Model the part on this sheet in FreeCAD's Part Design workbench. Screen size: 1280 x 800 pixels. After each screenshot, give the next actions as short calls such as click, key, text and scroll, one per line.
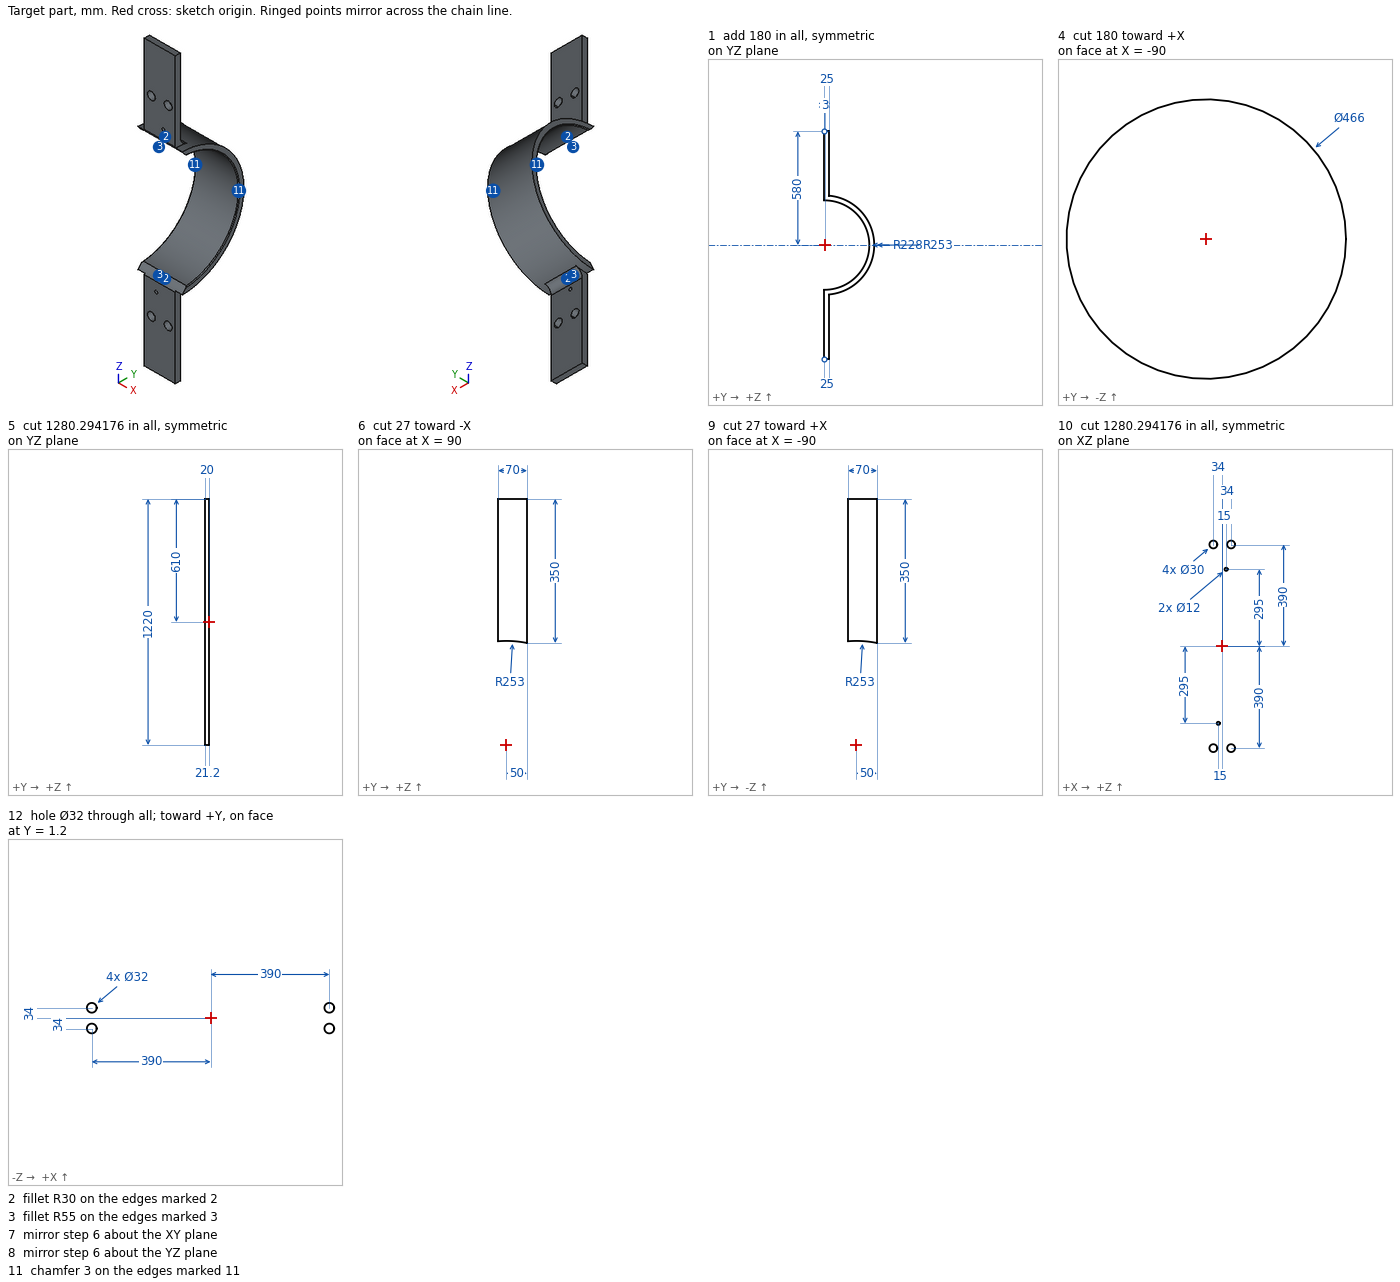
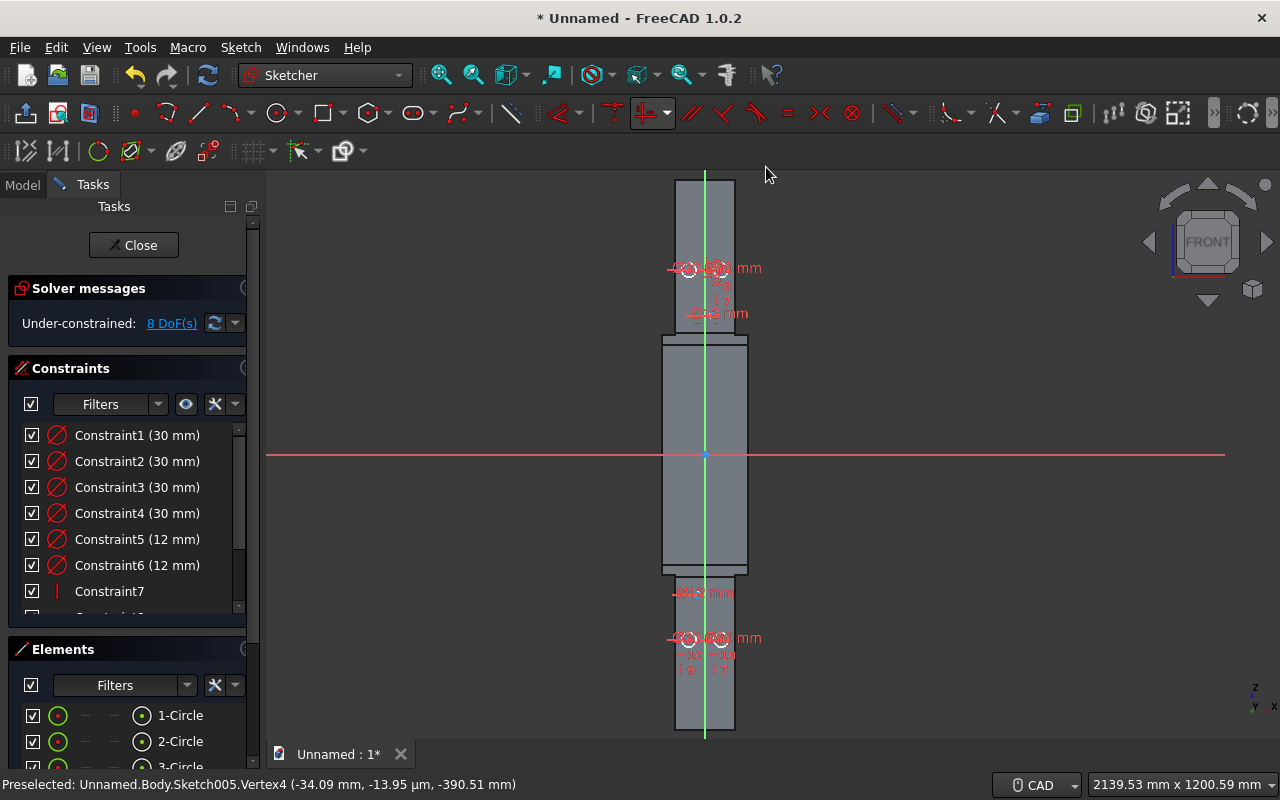
click(558, 114)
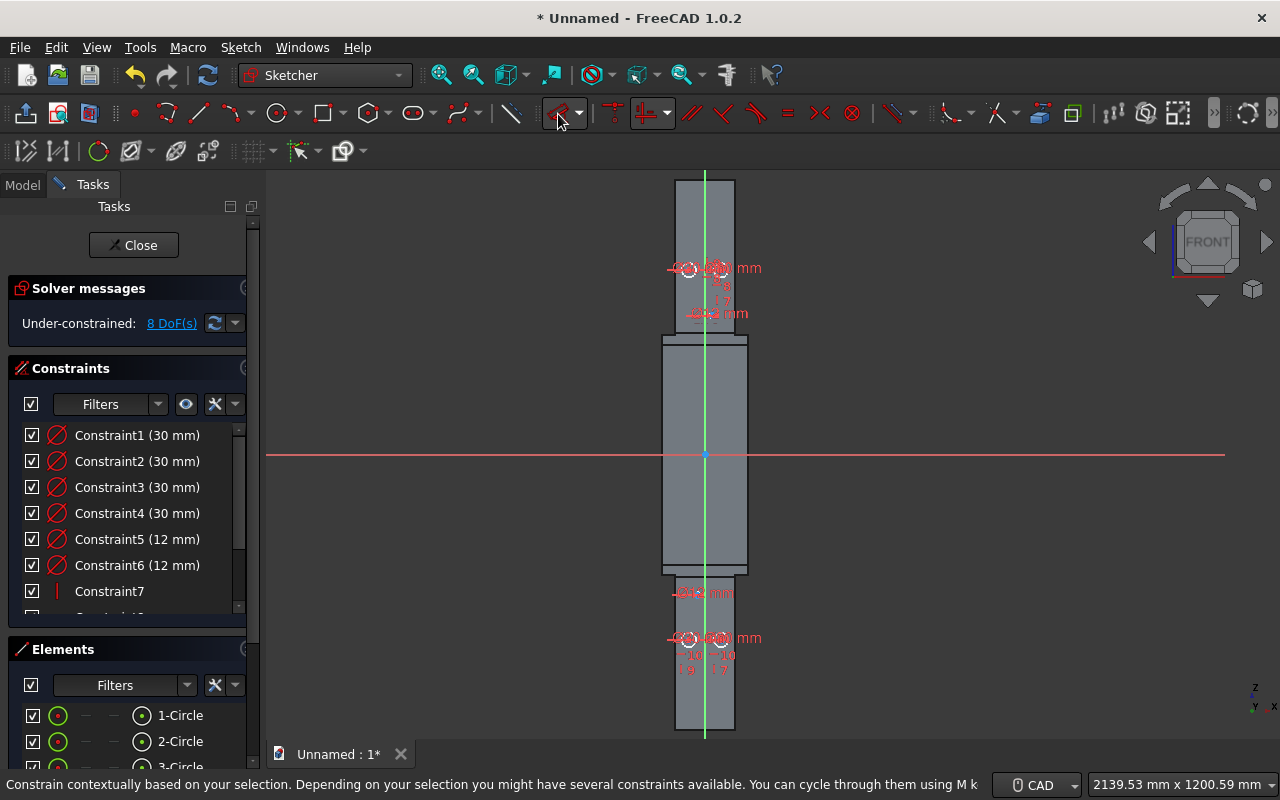
scroll(721, 270, up, 5)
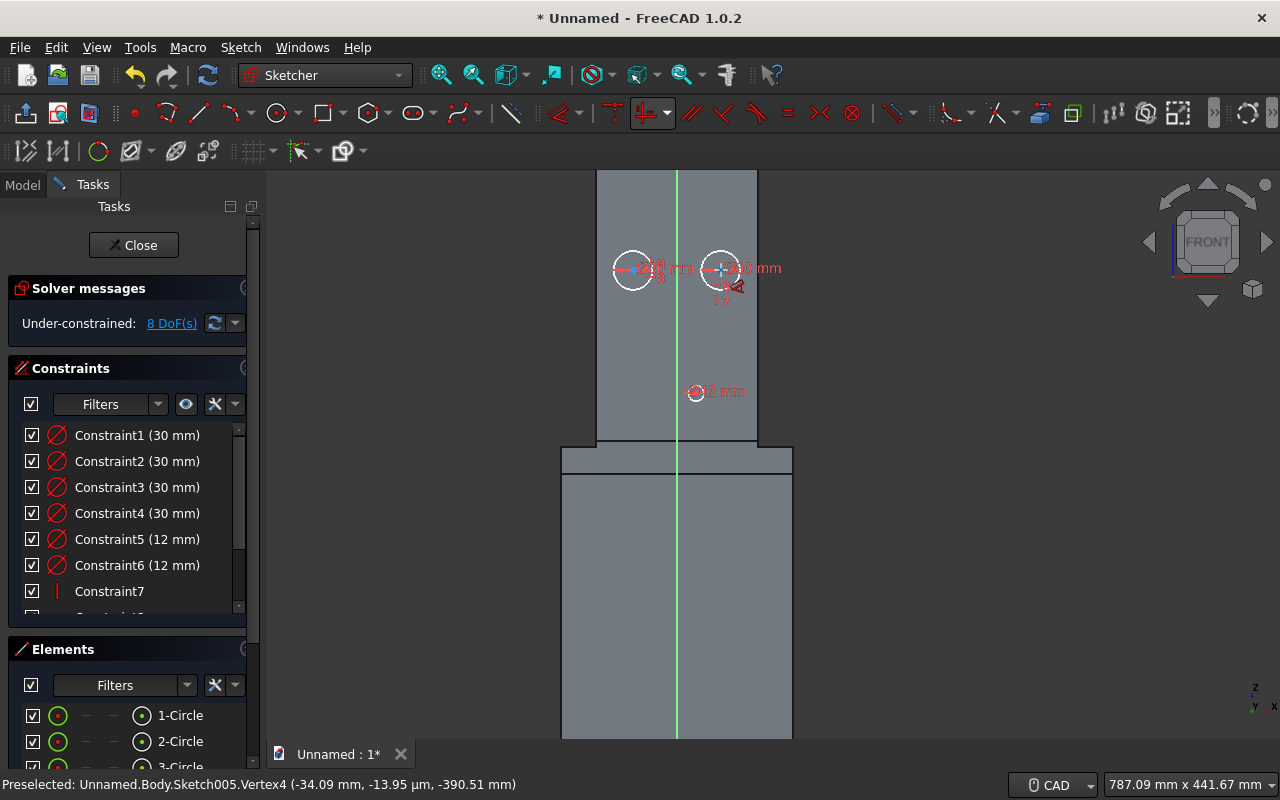
click(721, 270)
click(699, 236)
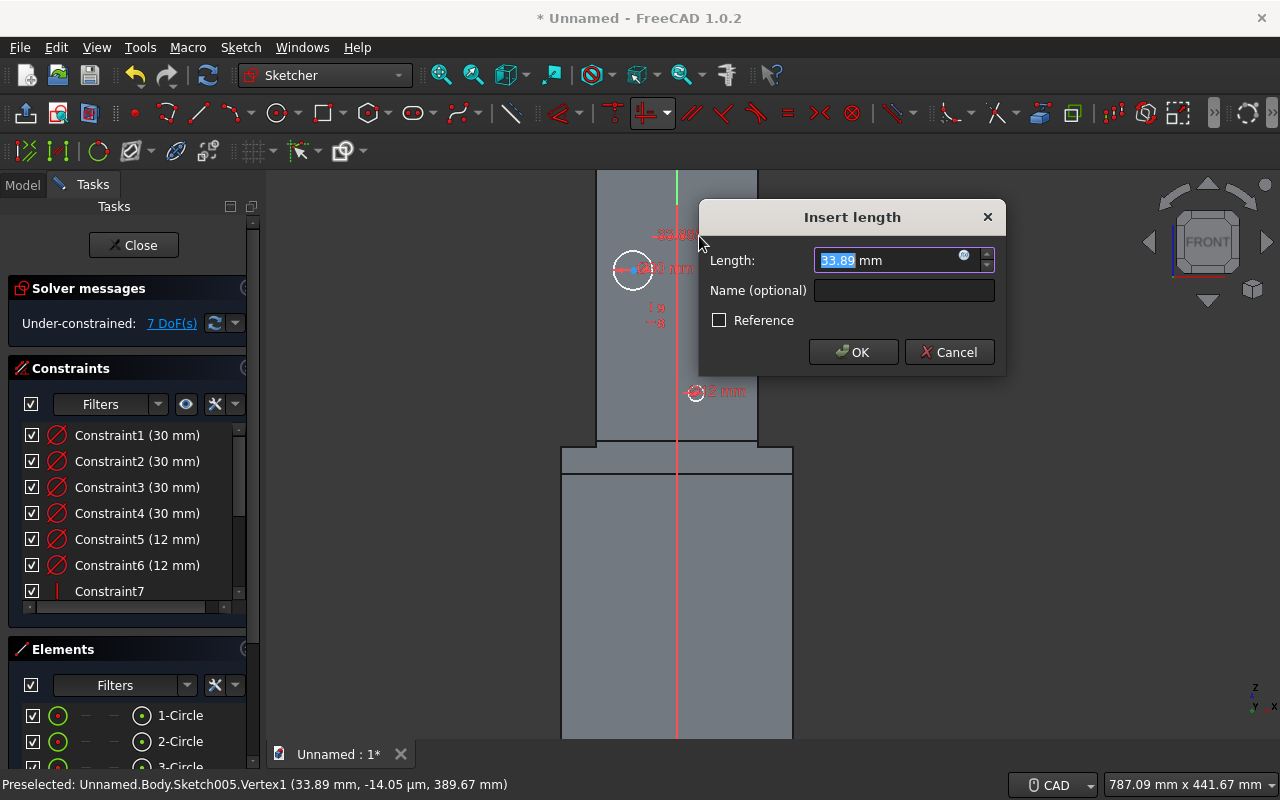
text(34)
key(Return)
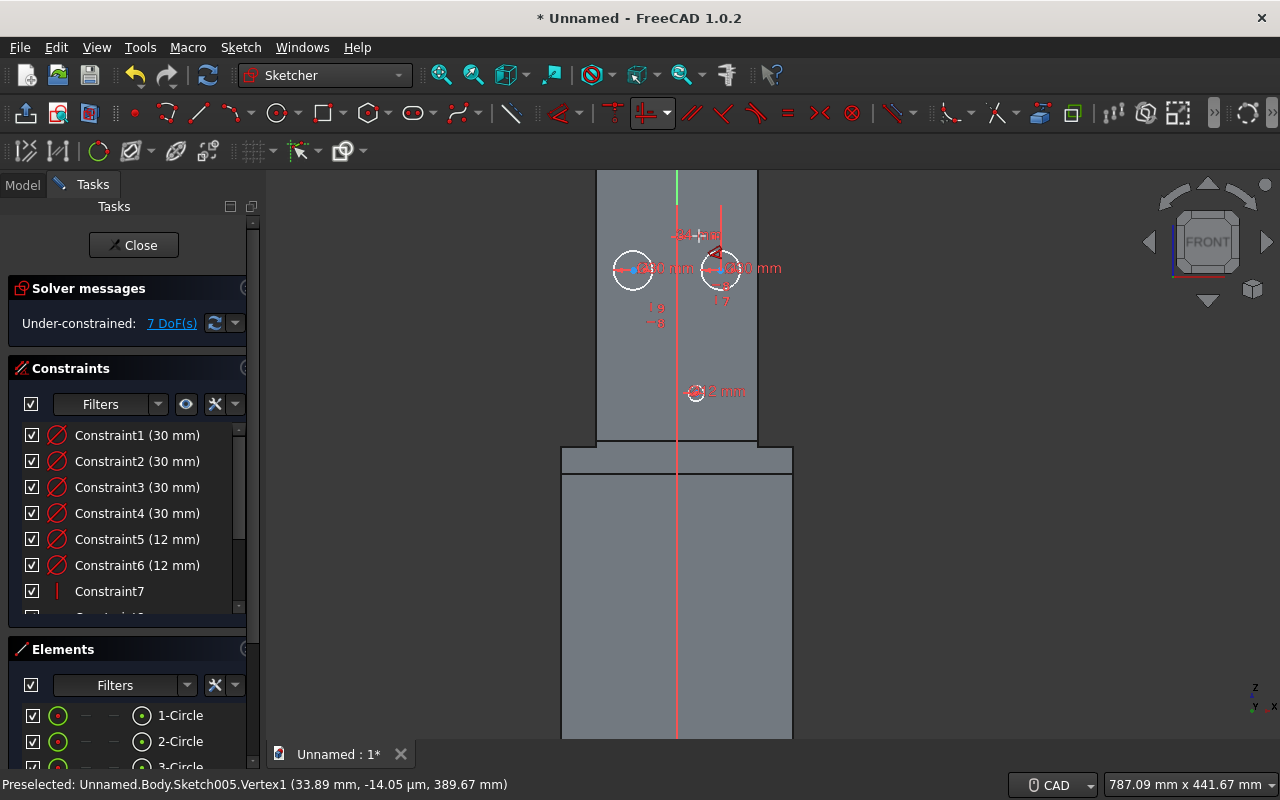
click(633, 270)
click(655, 212)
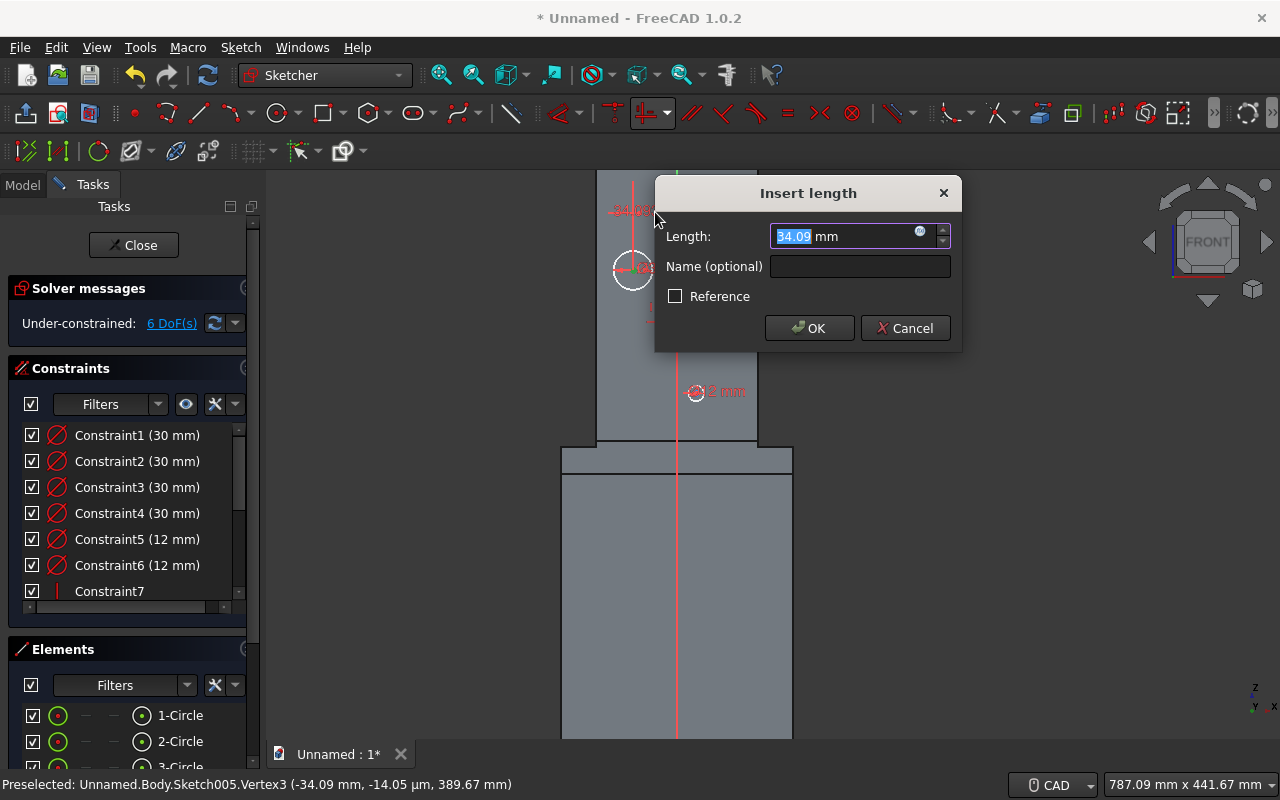
text(34)
key(Return)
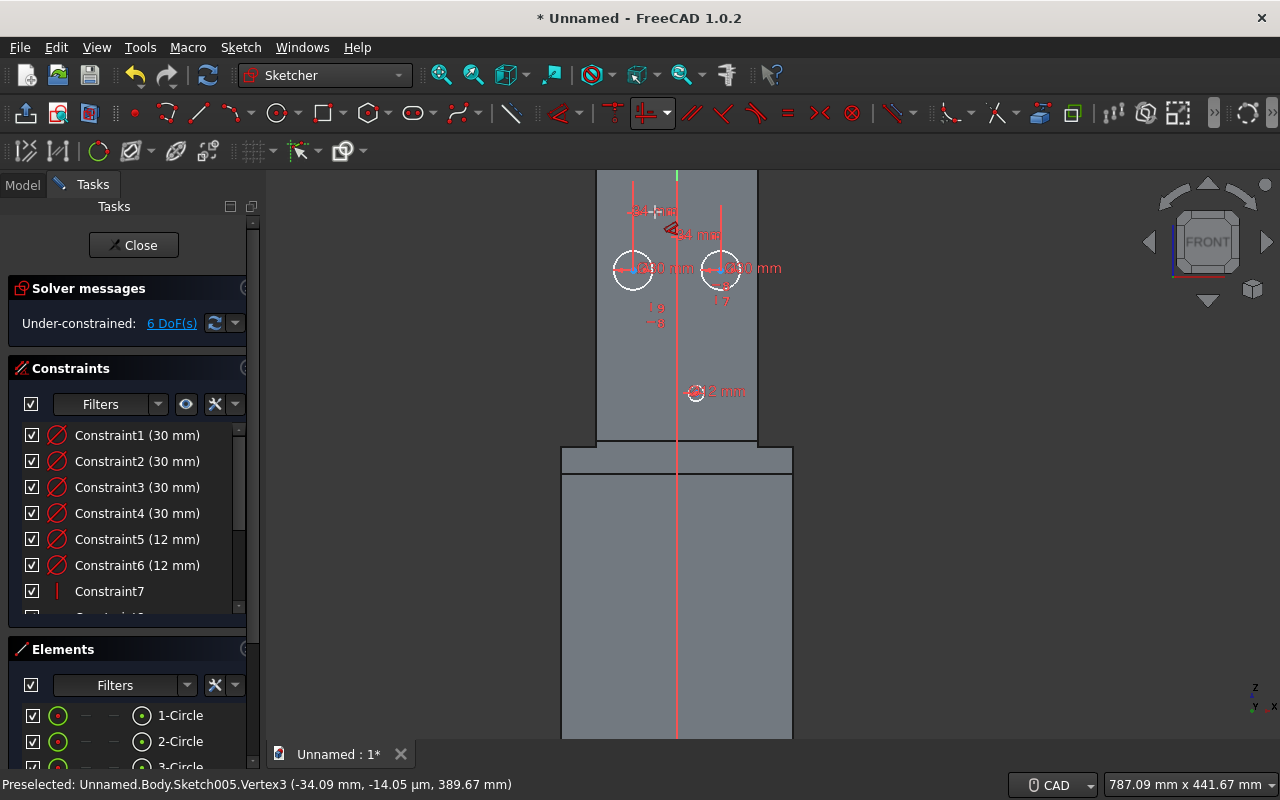
scroll(696, 393, up, 4)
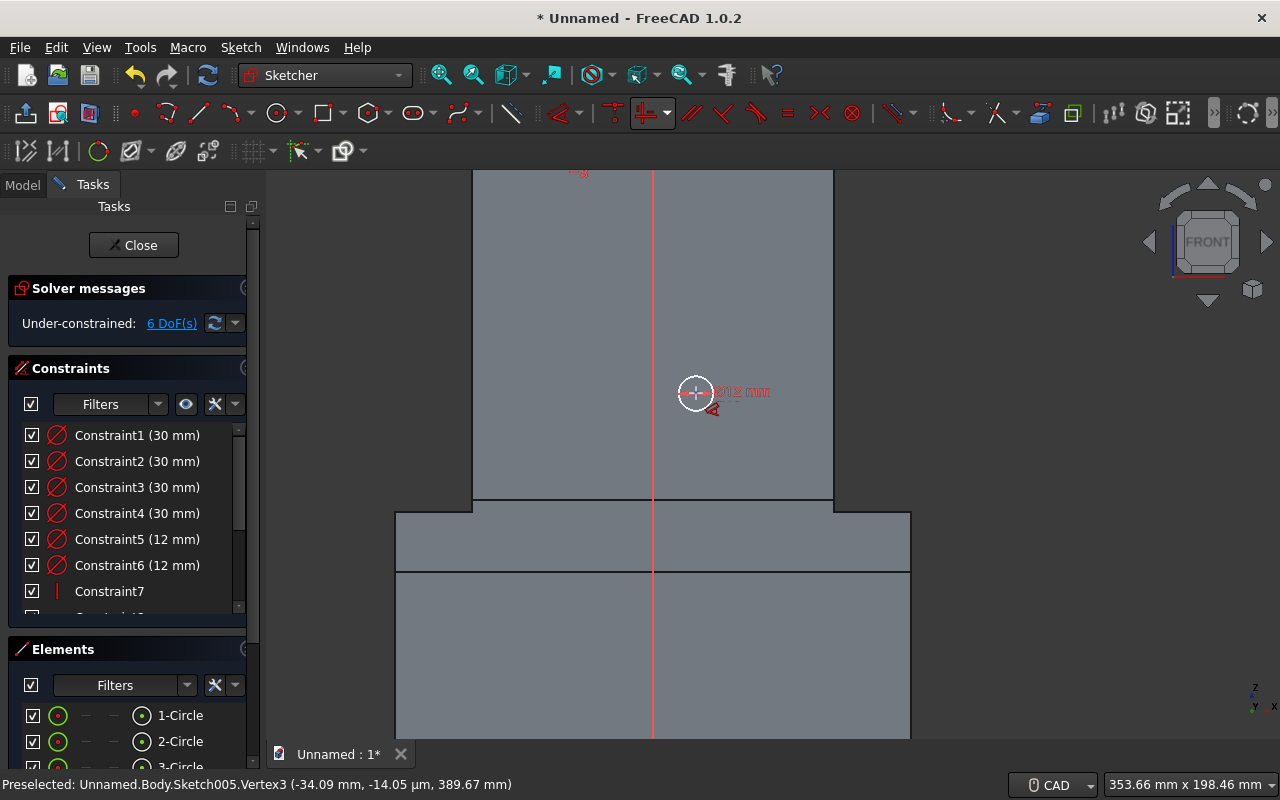
click(696, 394)
click(675, 360)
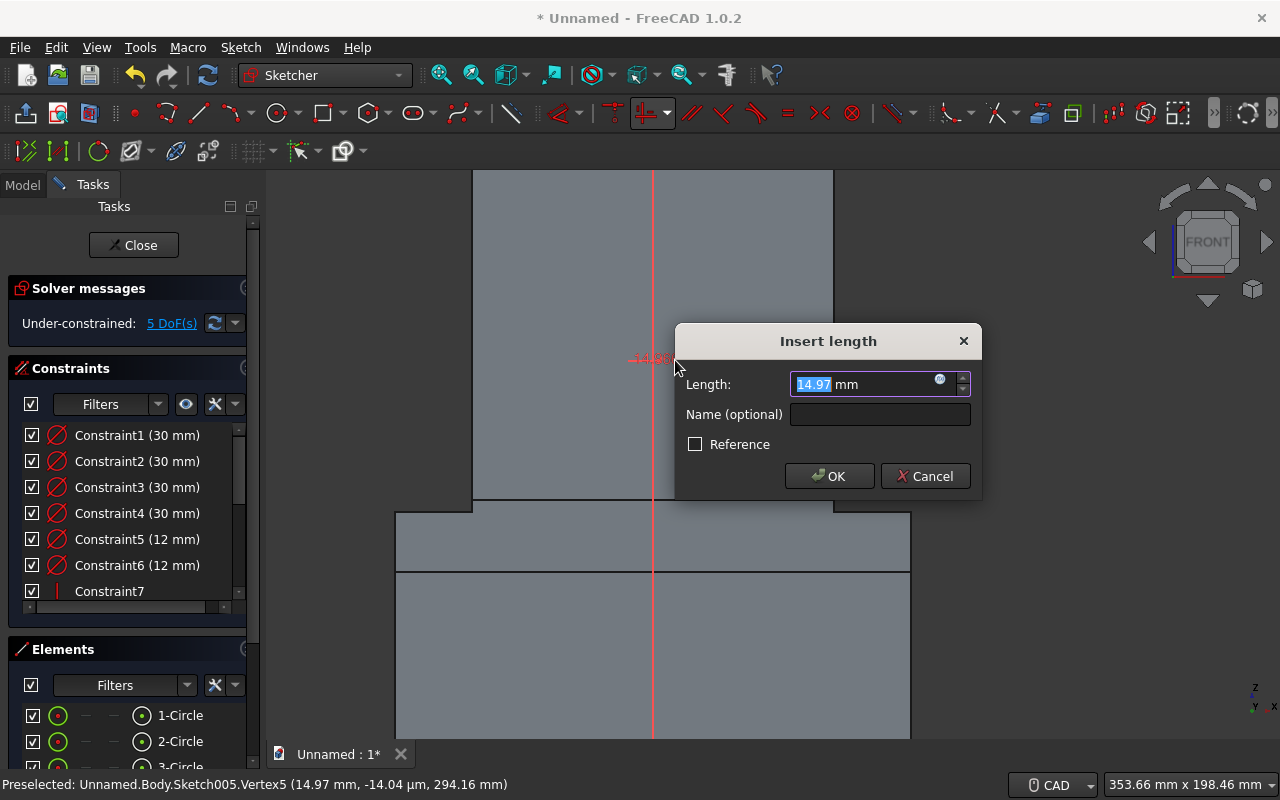
text(15)
key(Return)